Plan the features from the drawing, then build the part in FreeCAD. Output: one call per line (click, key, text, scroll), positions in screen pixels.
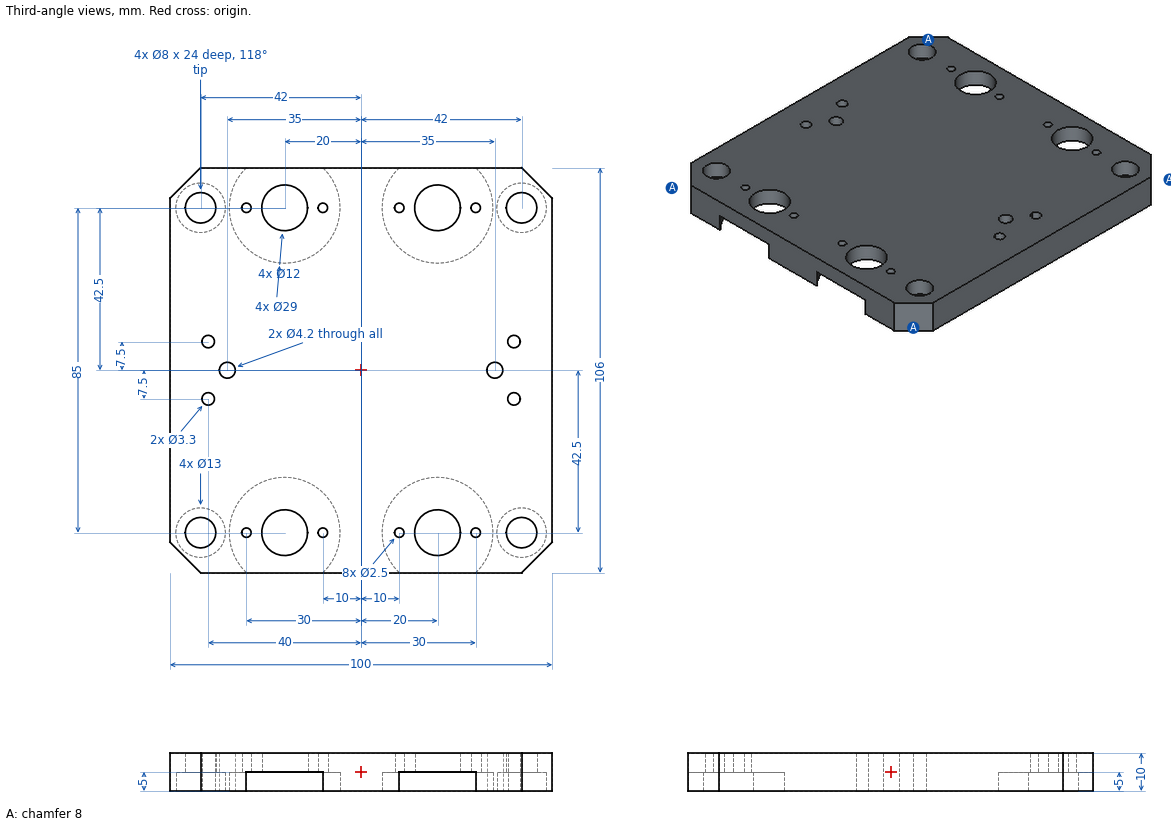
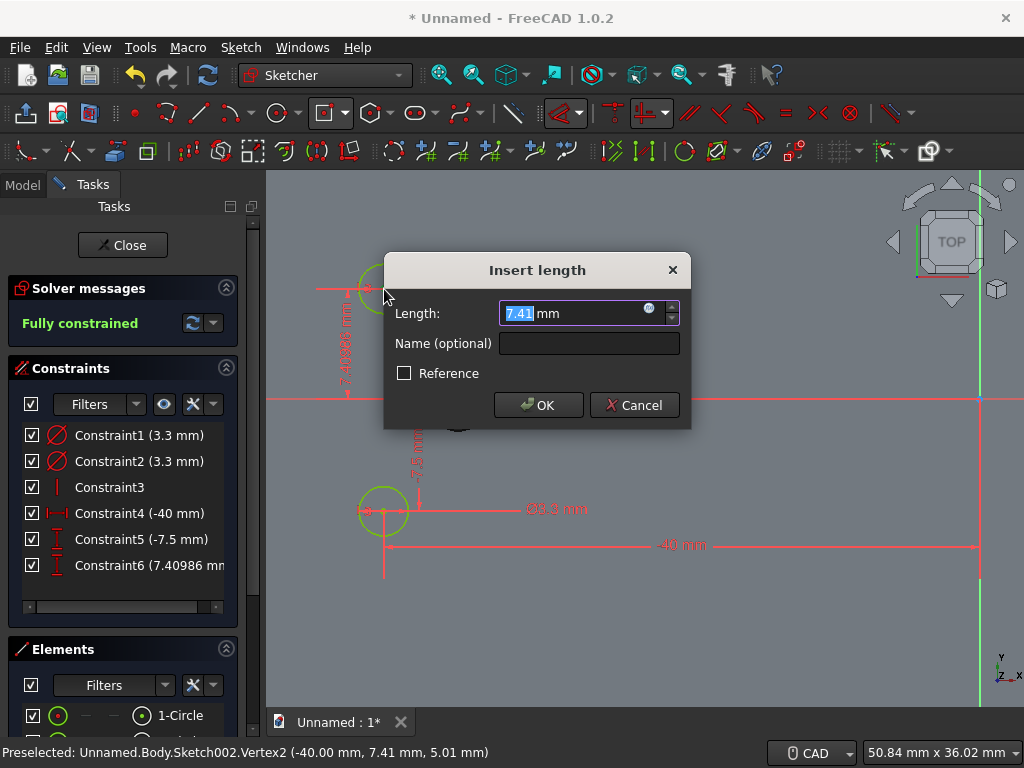
text(7.5)
key(Return)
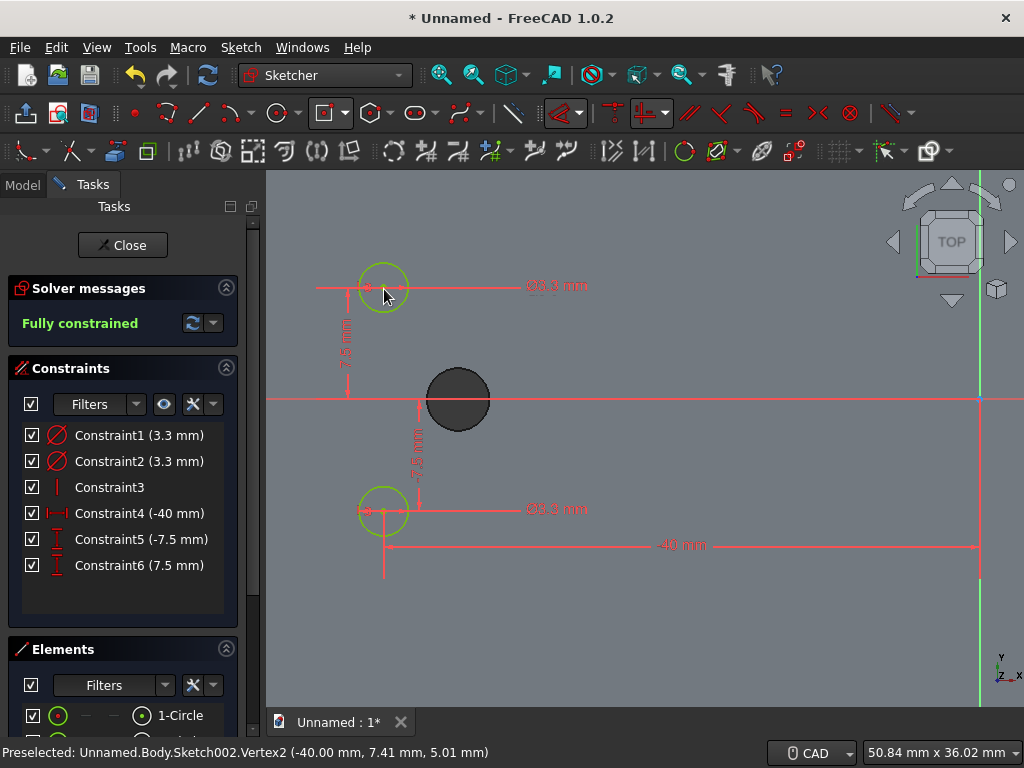
click(123, 245)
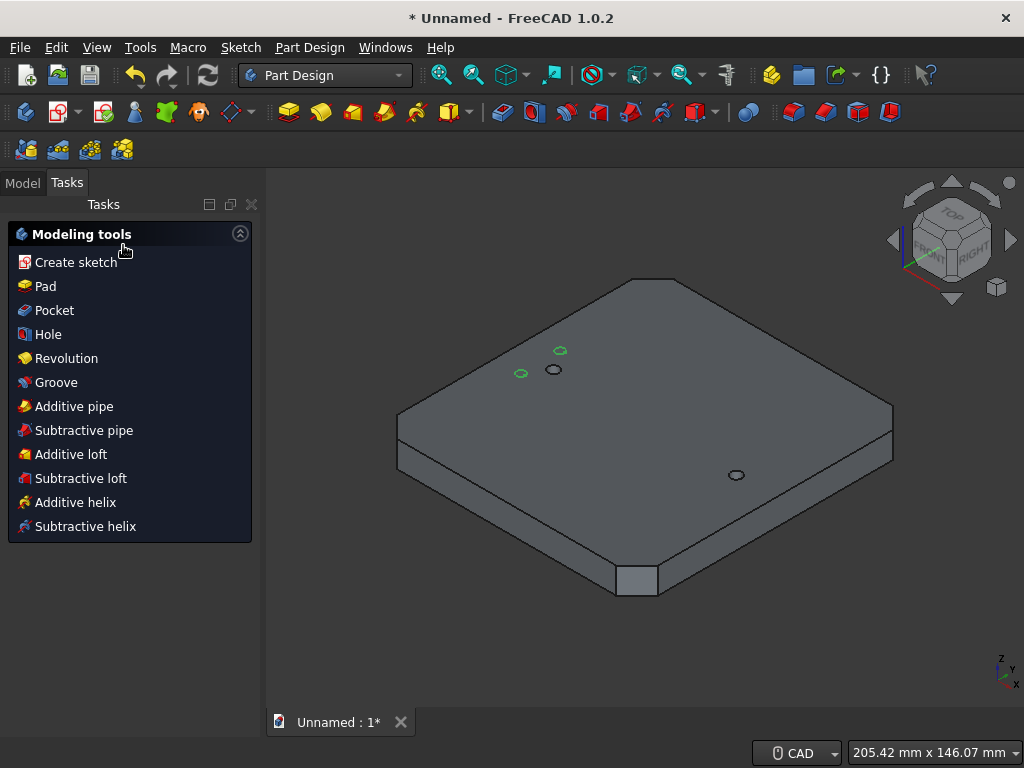
click(504, 112)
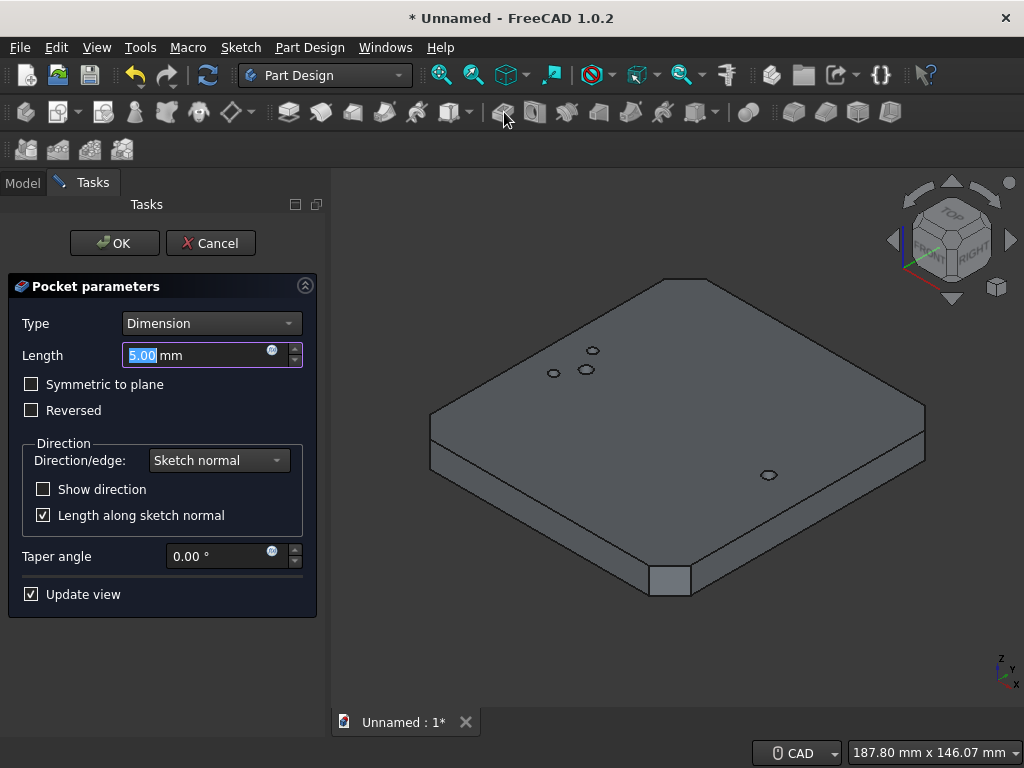
click(212, 324)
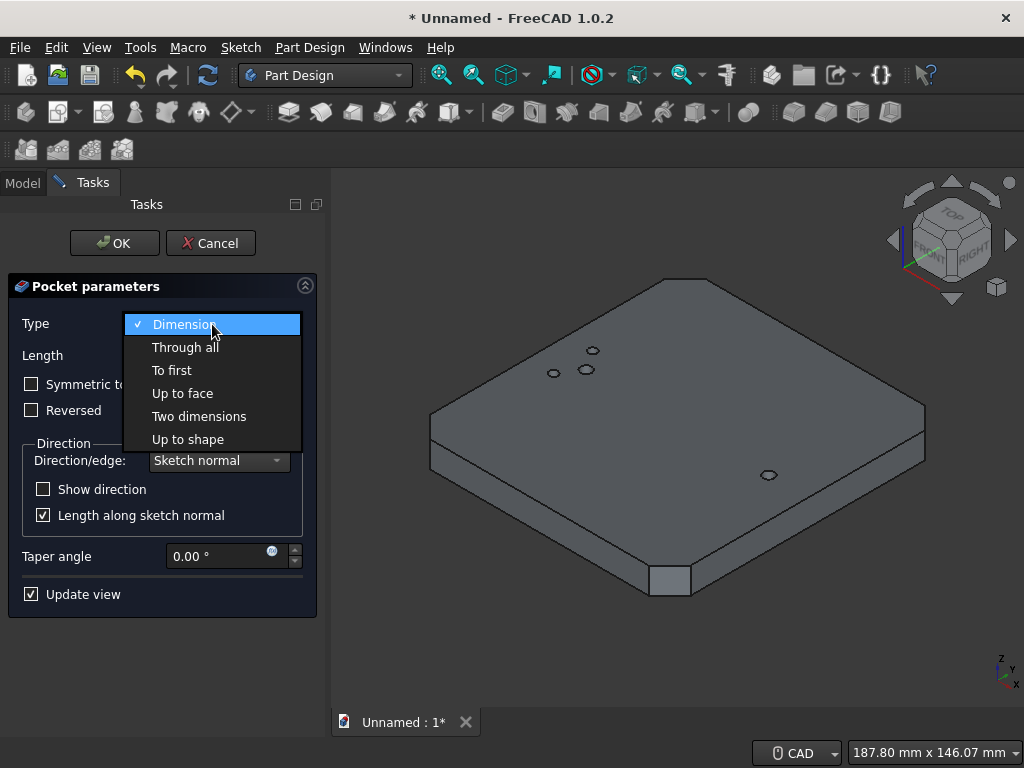
click(212, 348)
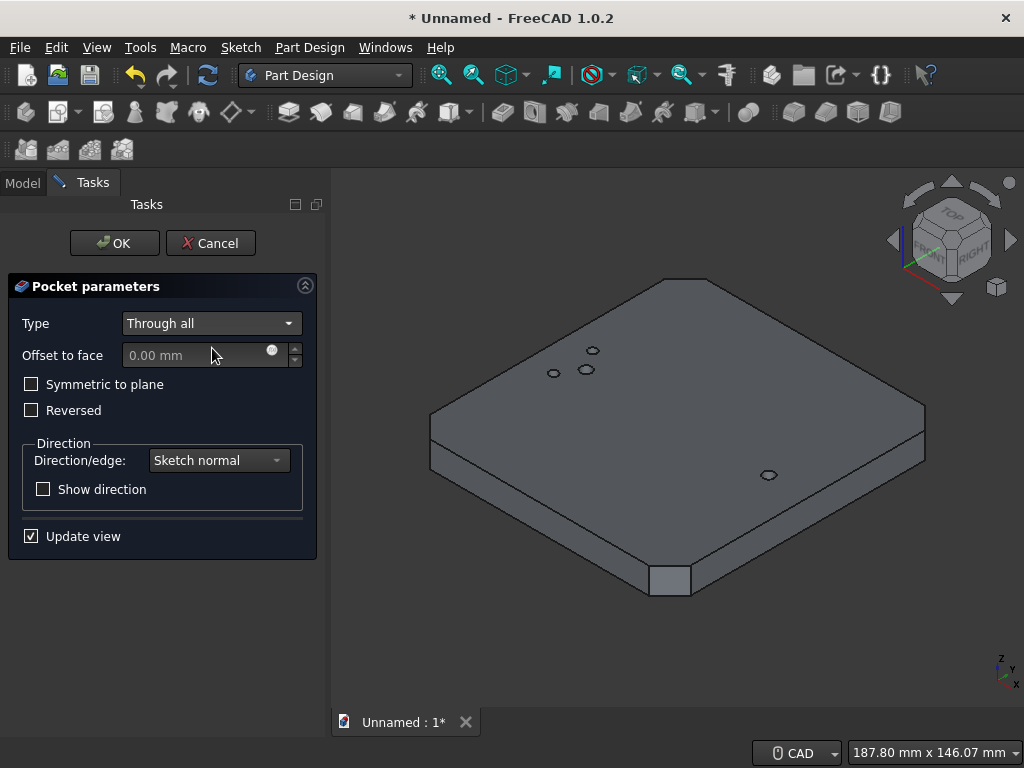
click(115, 243)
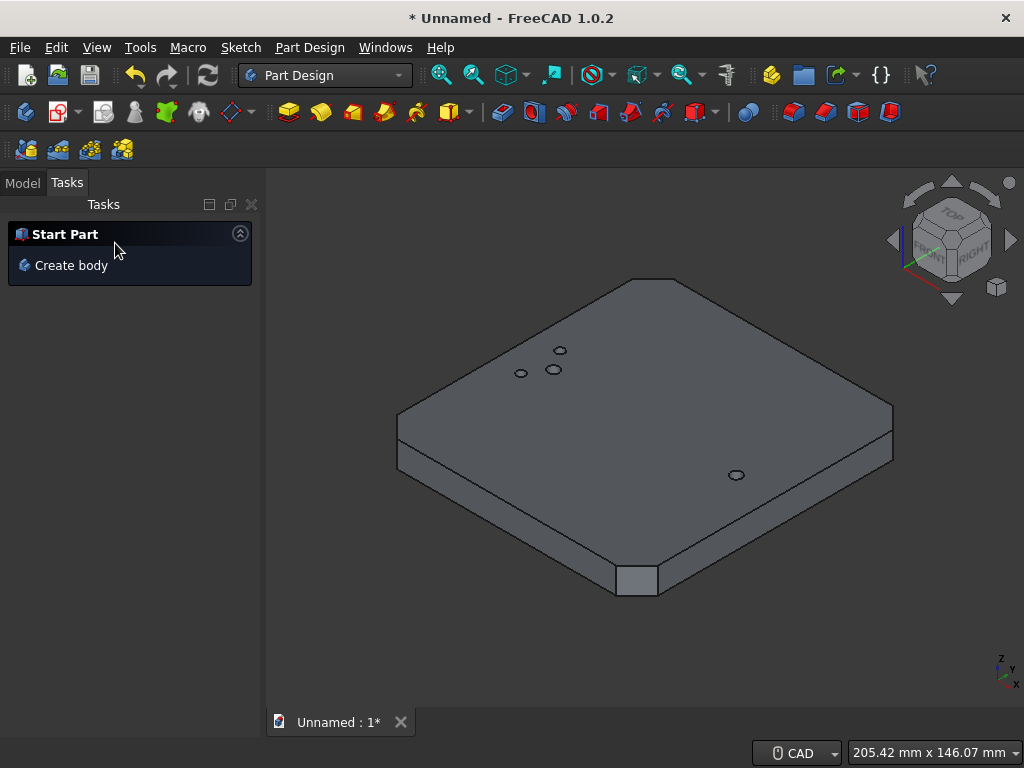
click(23, 182)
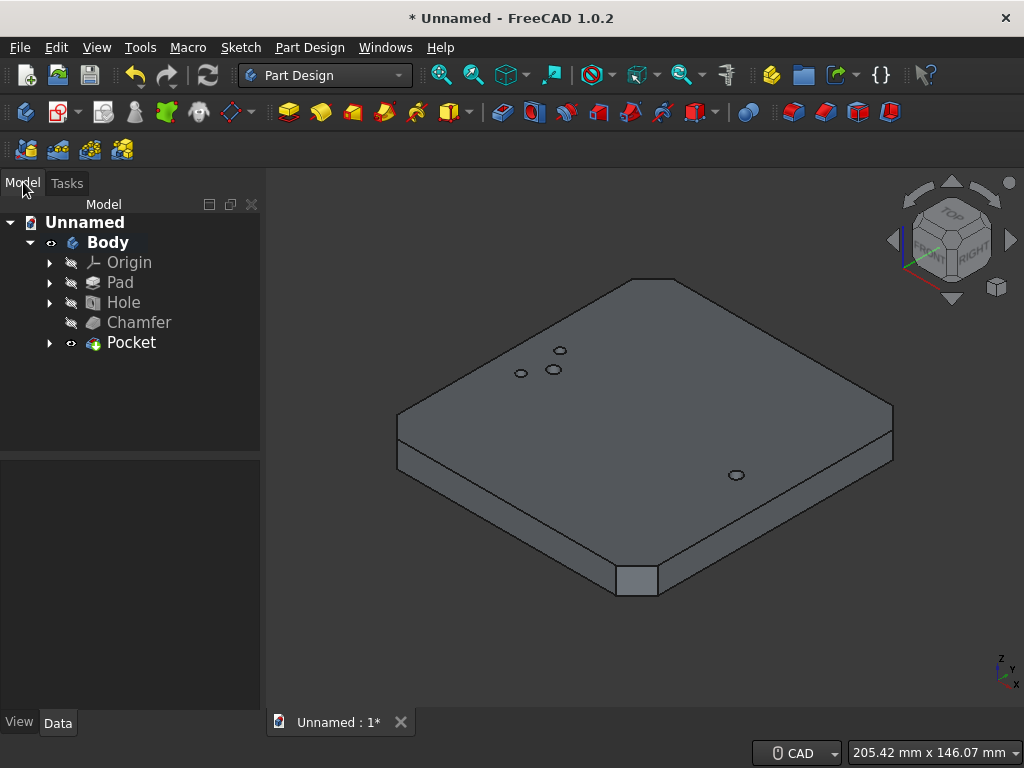
click(116, 343)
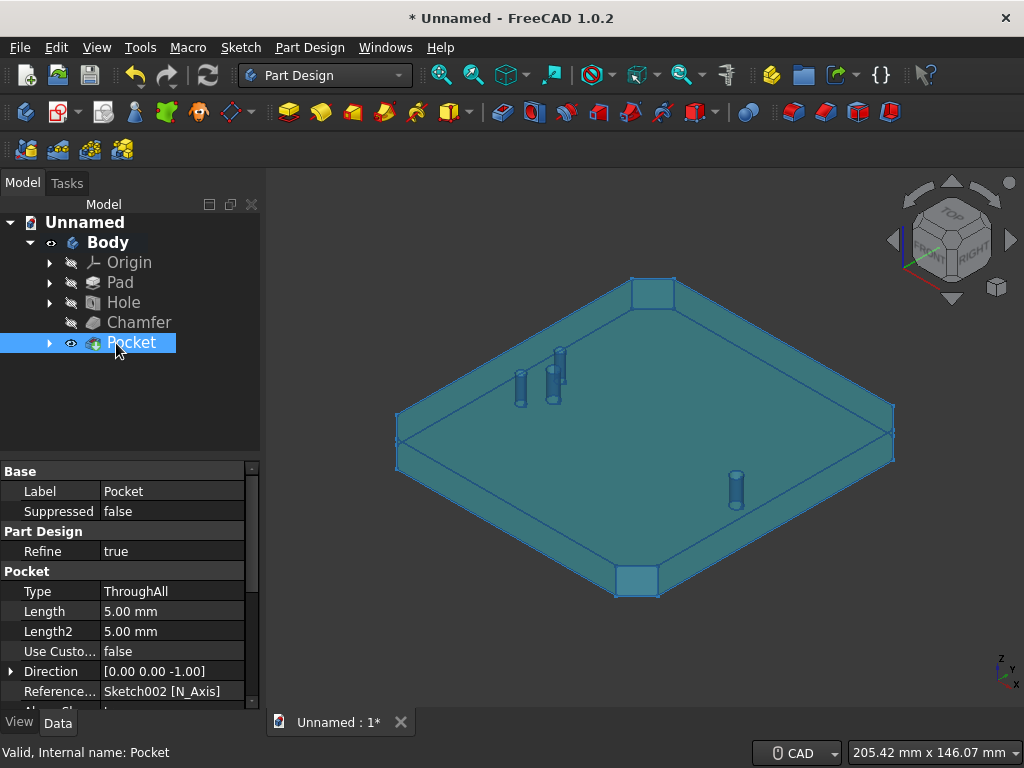
click(26, 150)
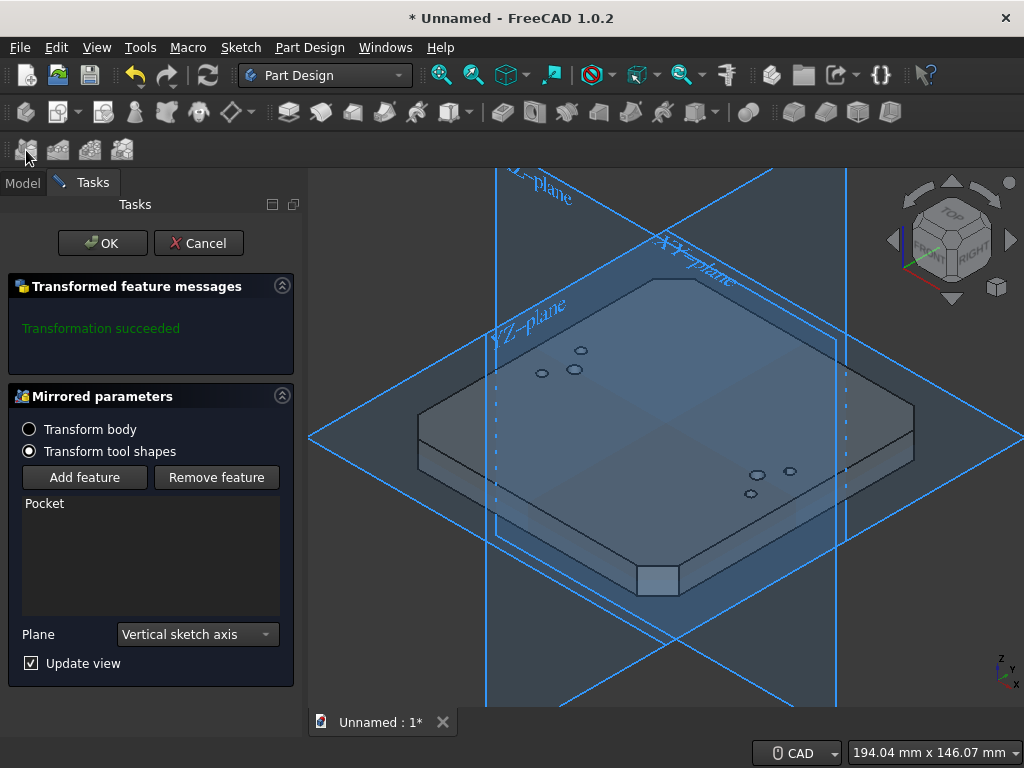
click(198, 634)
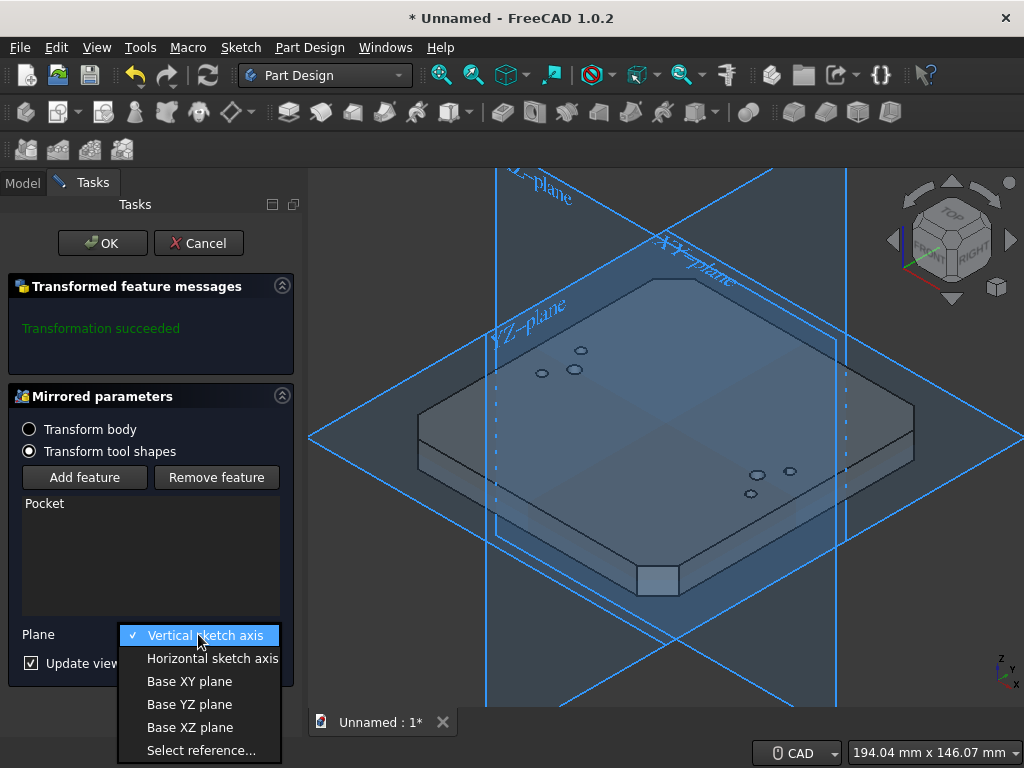
click(198, 704)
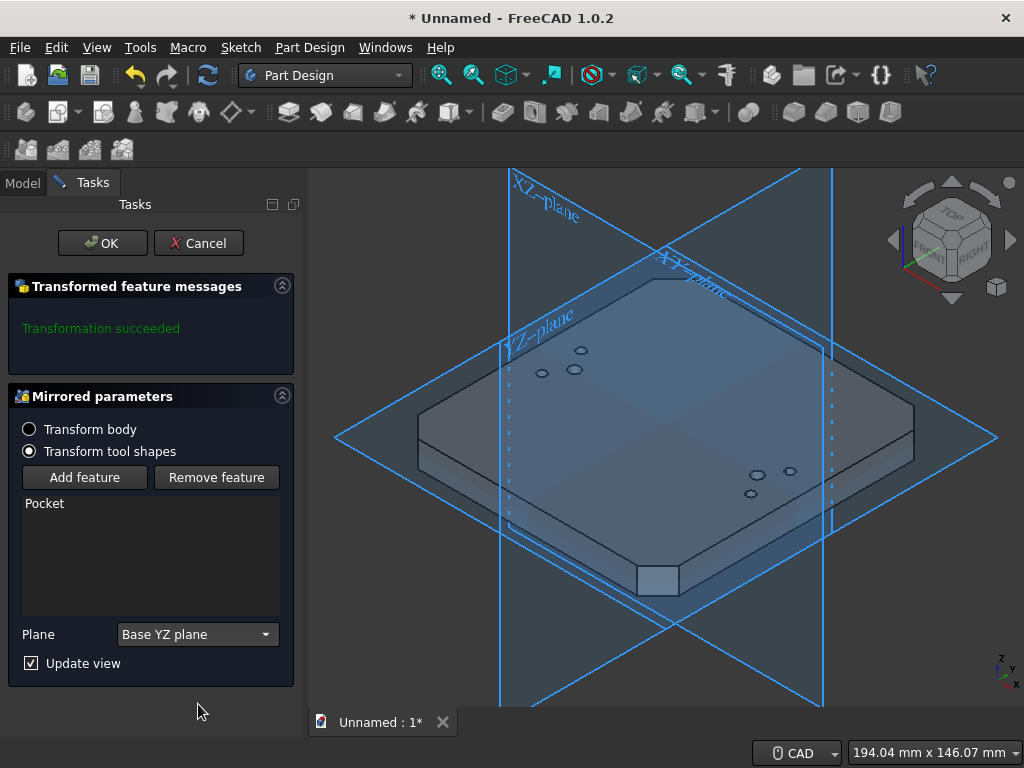
click(103, 243)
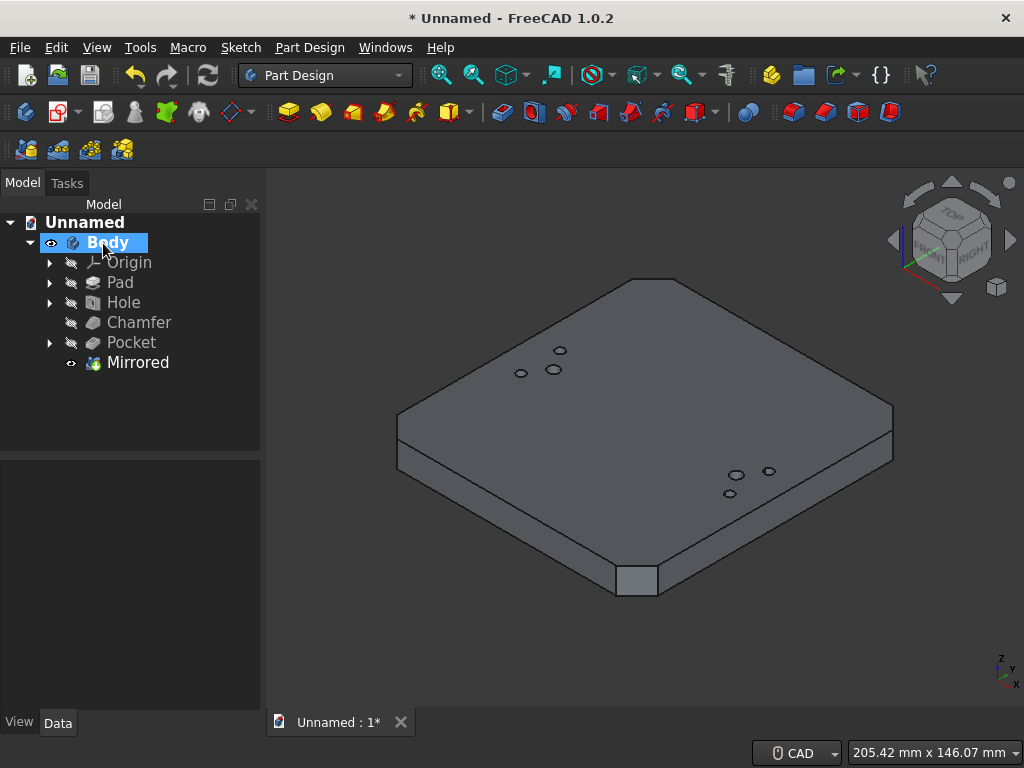
click(685, 399)